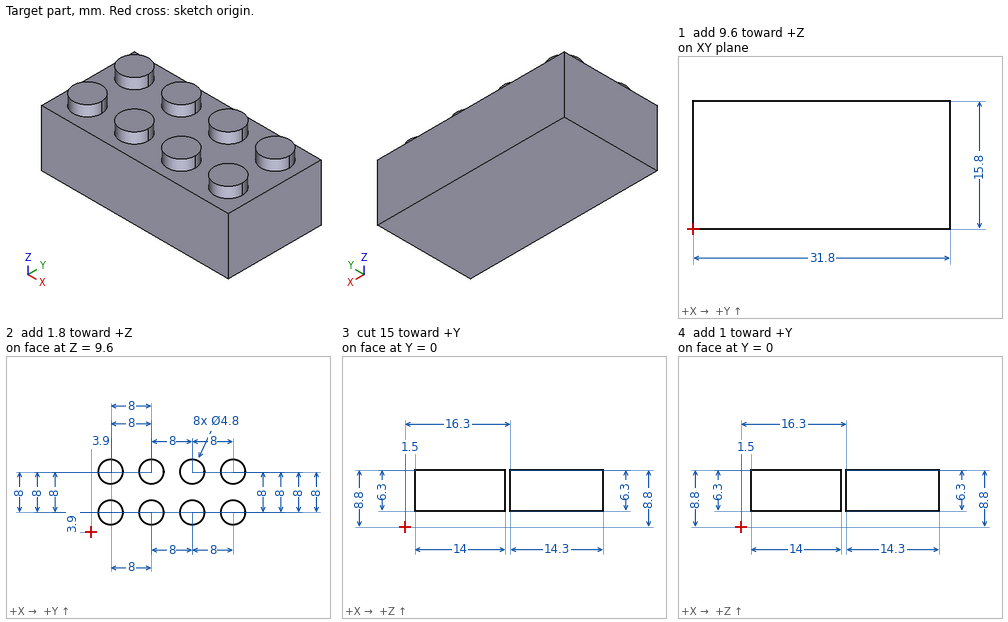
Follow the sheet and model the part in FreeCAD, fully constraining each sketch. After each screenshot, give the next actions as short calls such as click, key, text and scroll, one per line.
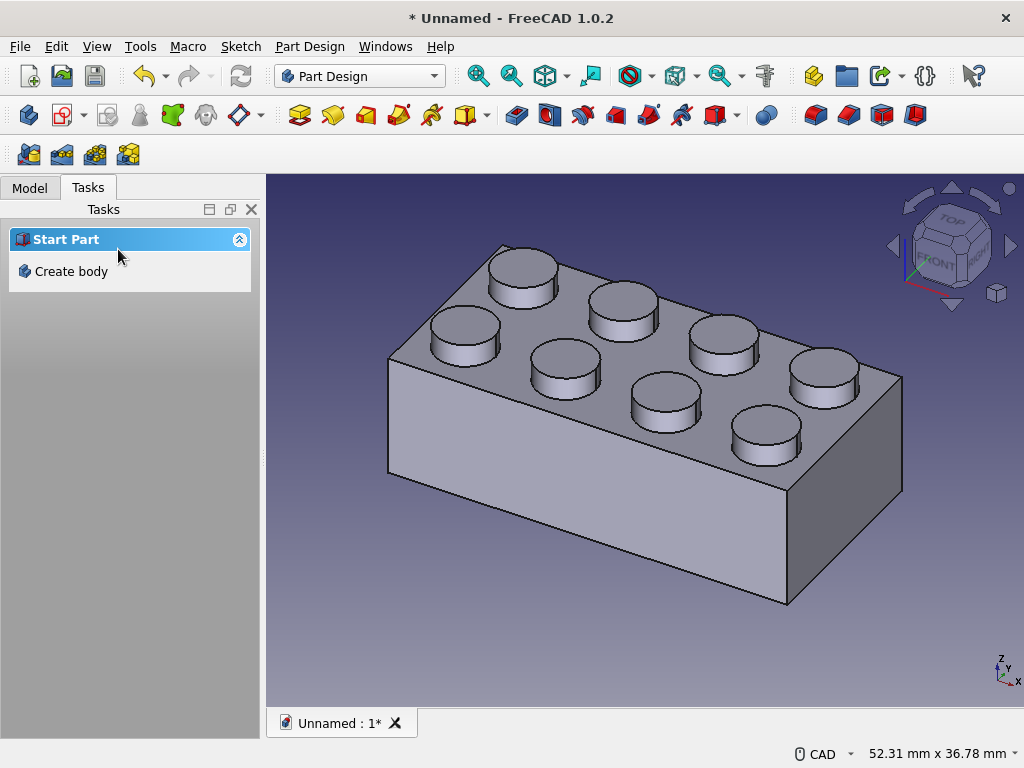
click(702, 519)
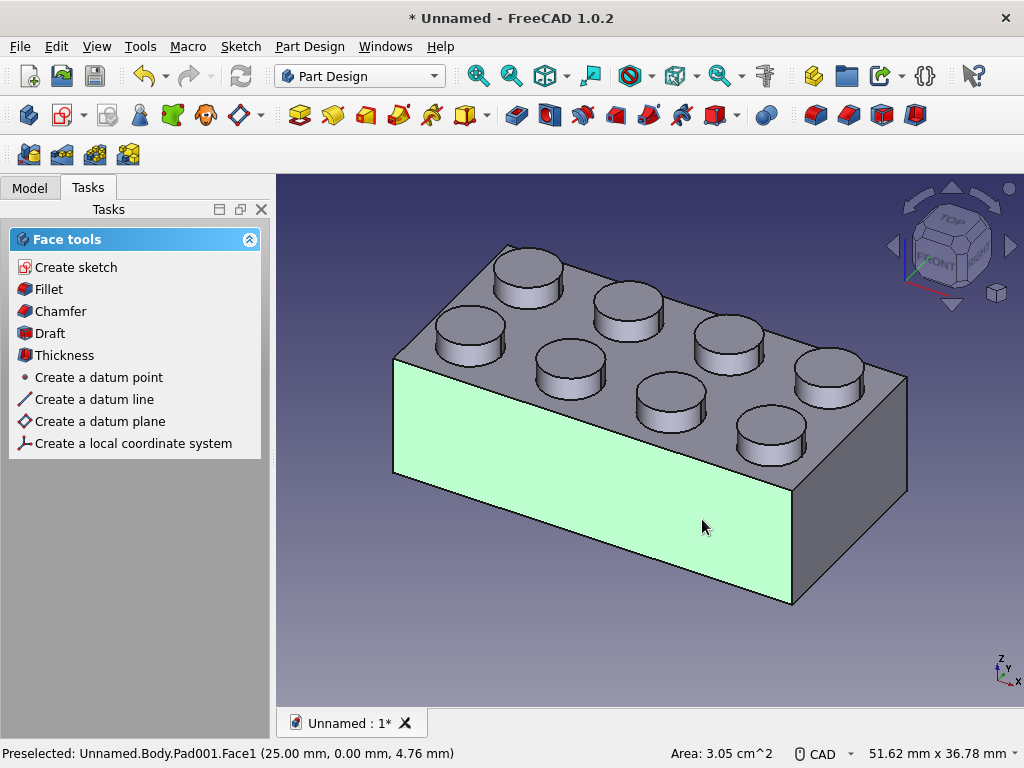
click(62, 116)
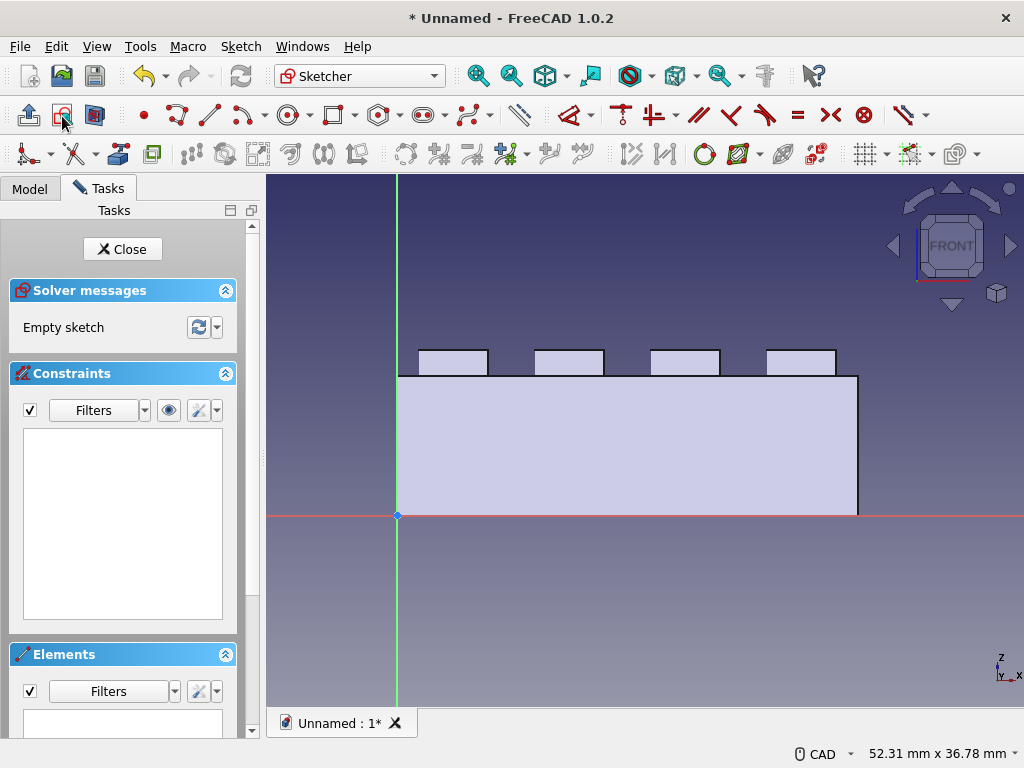
scroll(385, 390, down, 1)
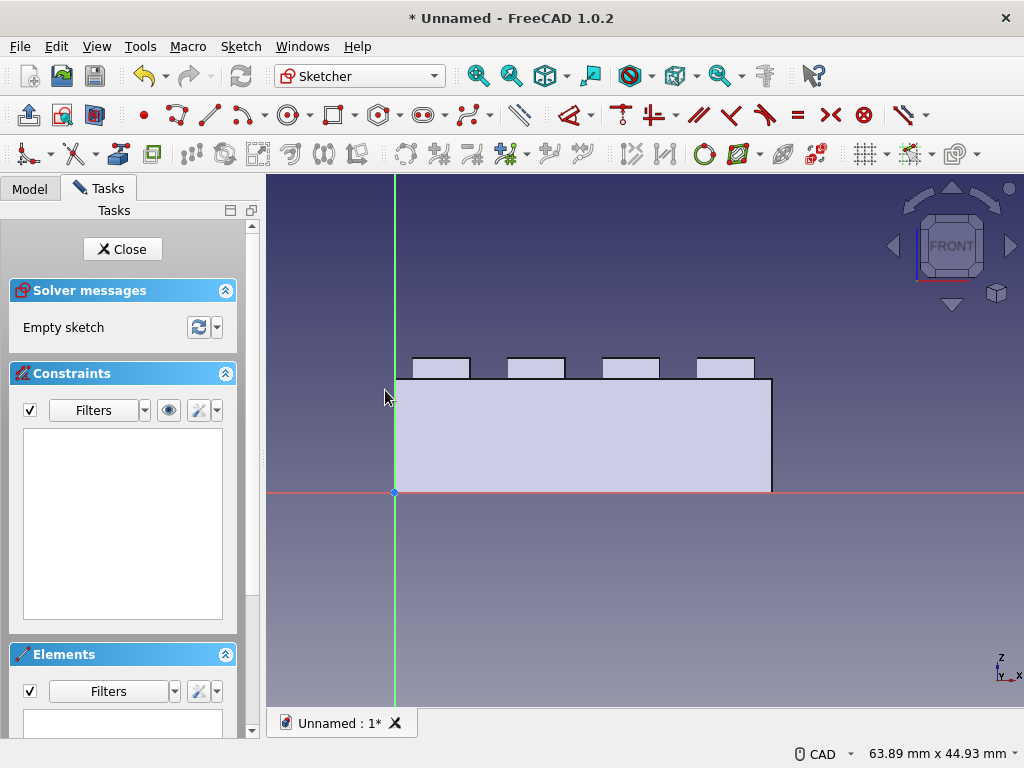
key(g)
key(r)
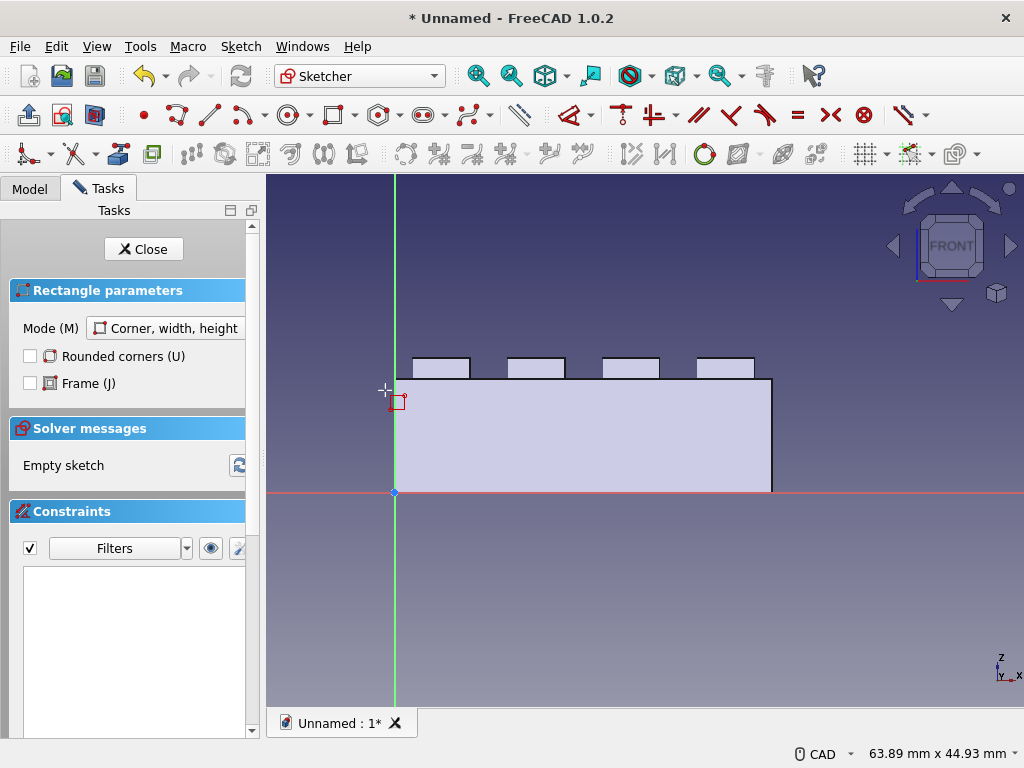
click(413, 388)
click(579, 463)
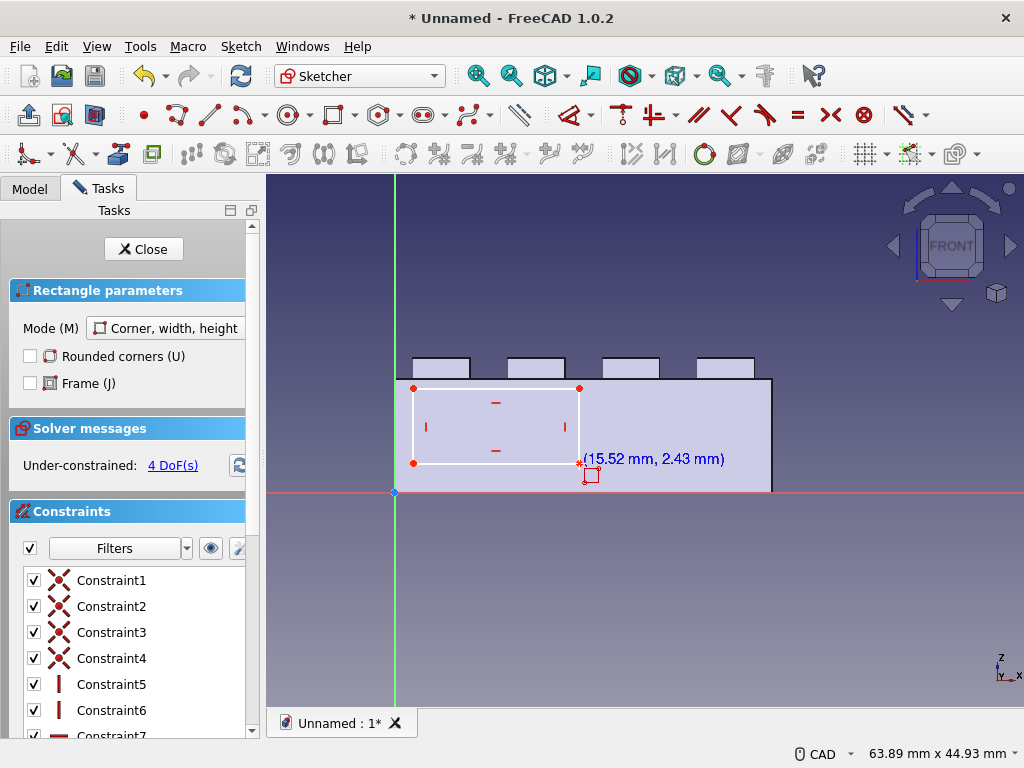
scroll(588, 388, up, 3)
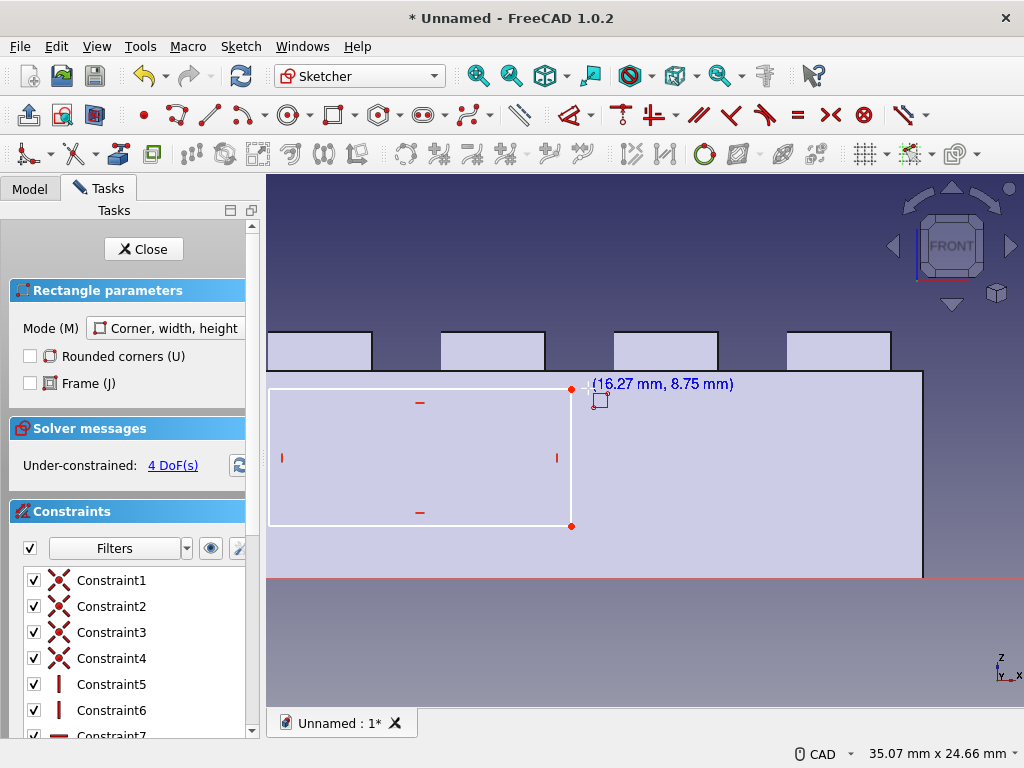
click(588, 388)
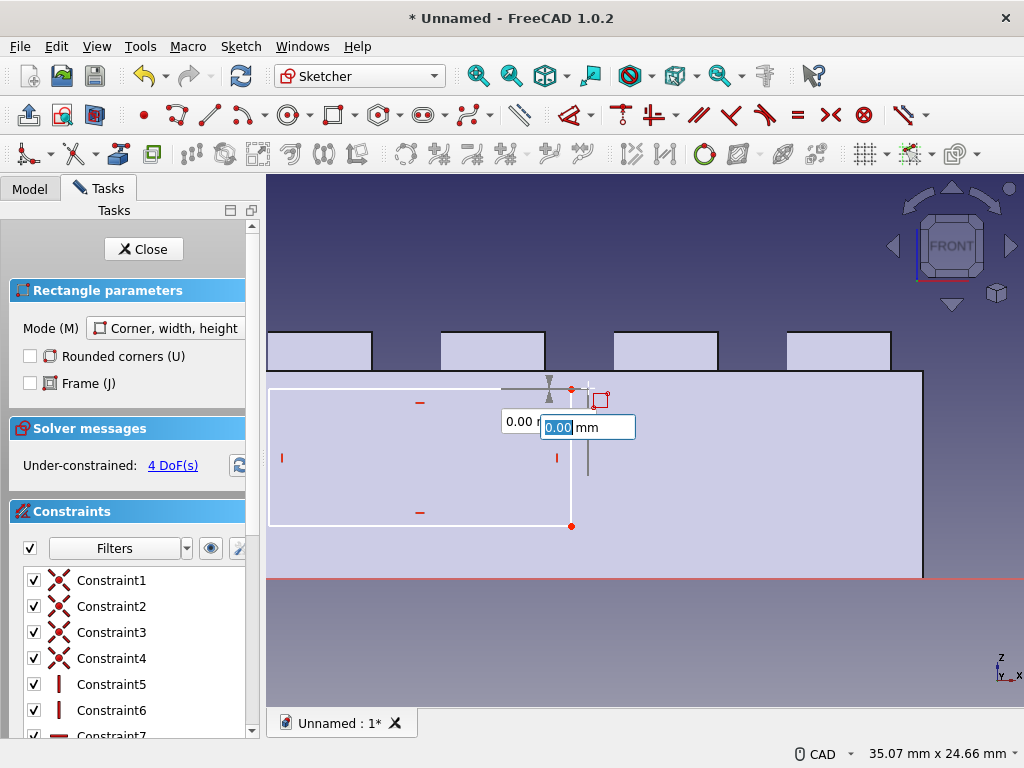
scroll(589, 388, down, 3)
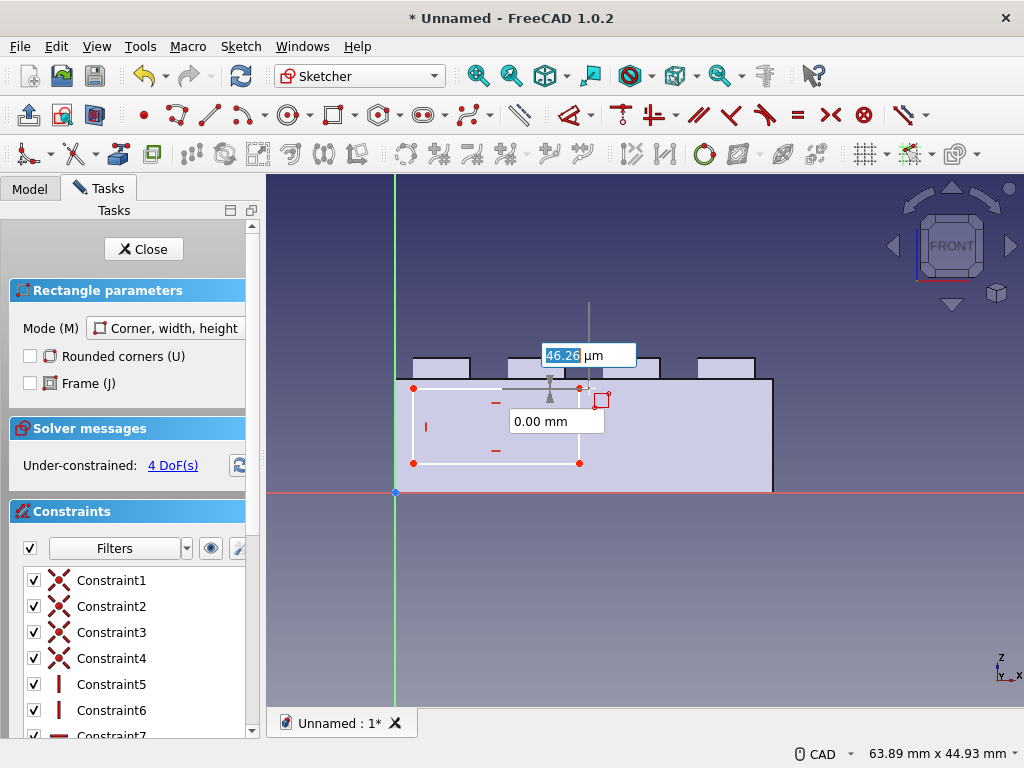
click(758, 463)
key(Escape)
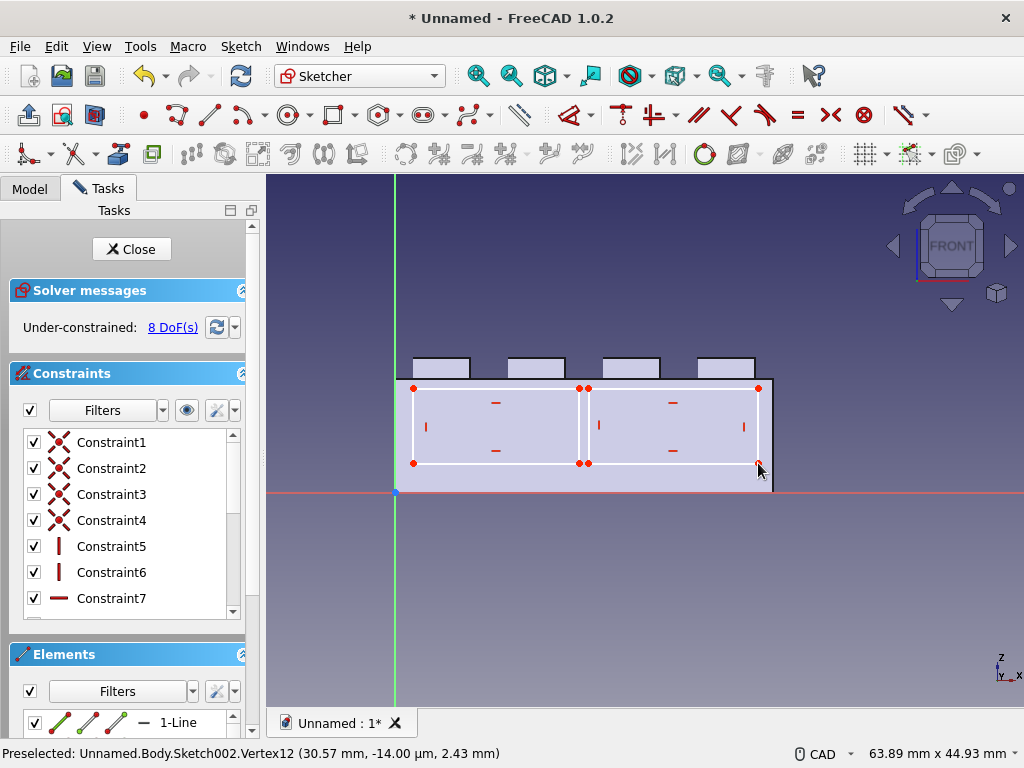
key(d)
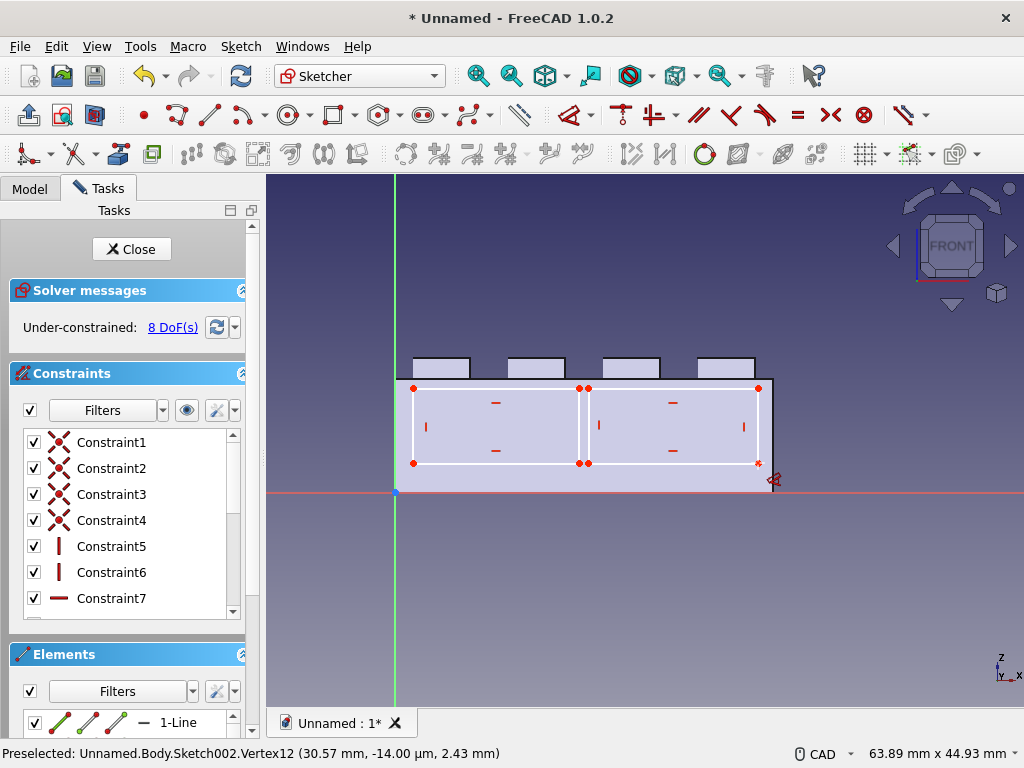
click(463, 464)
click(496, 430)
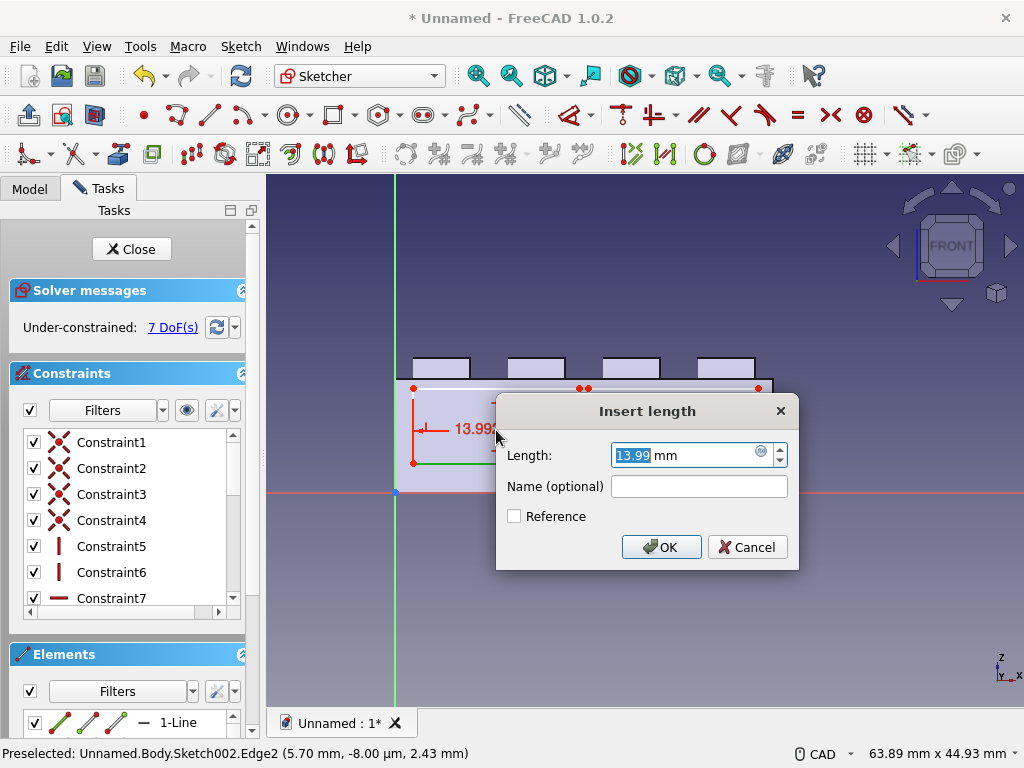
text(14)
key(Return)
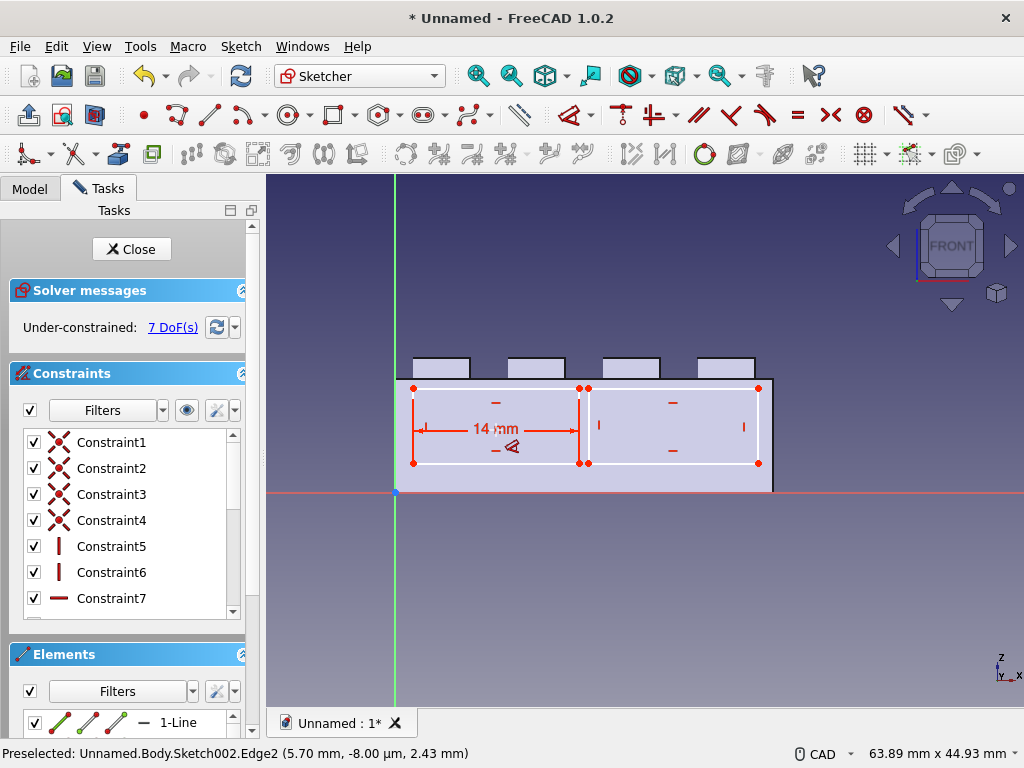
click(413, 411)
click(379, 426)